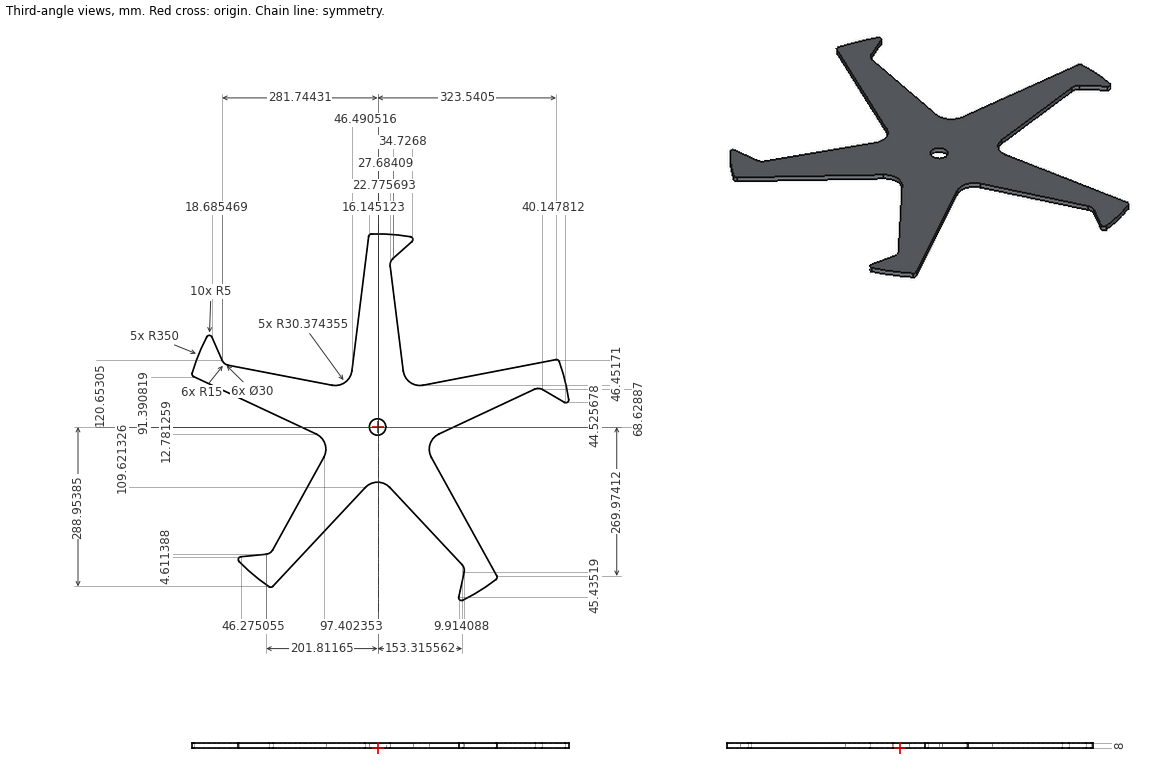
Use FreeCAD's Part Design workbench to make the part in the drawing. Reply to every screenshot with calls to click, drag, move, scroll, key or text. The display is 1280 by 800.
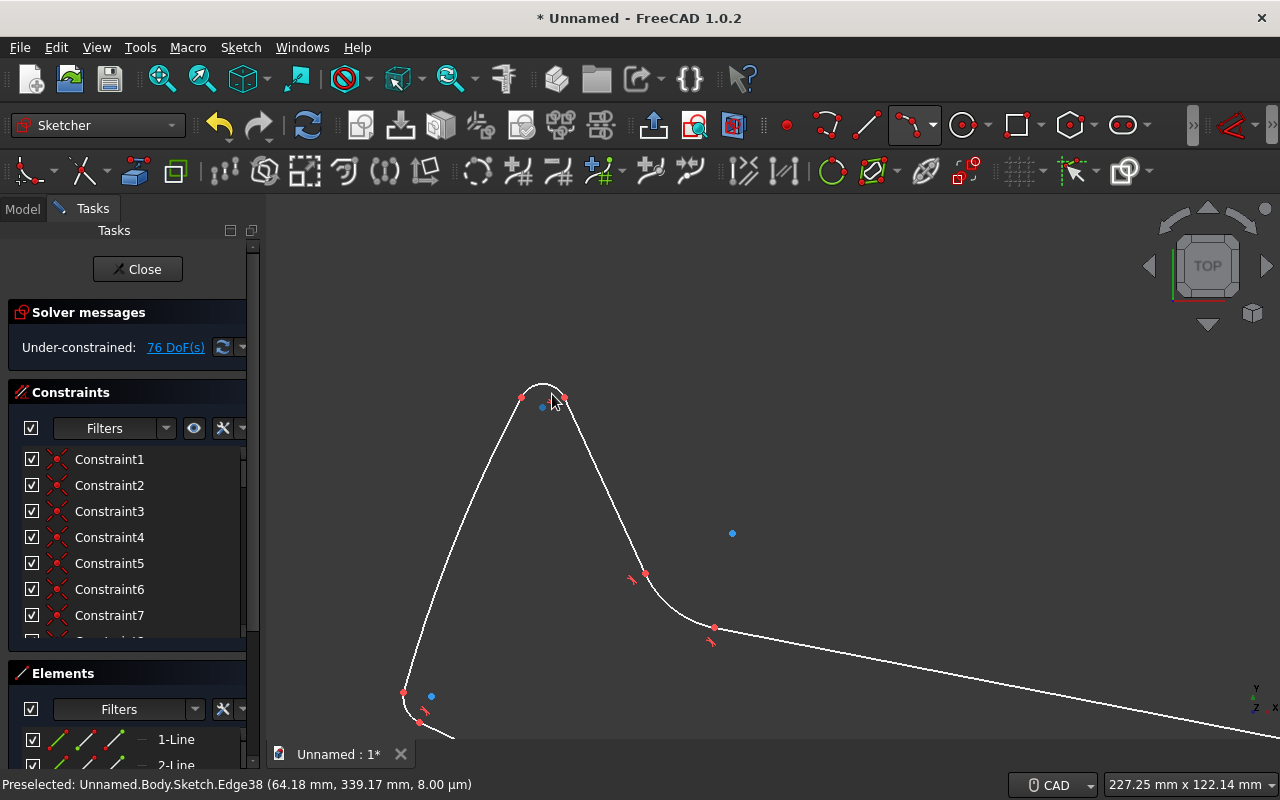
click(554, 387)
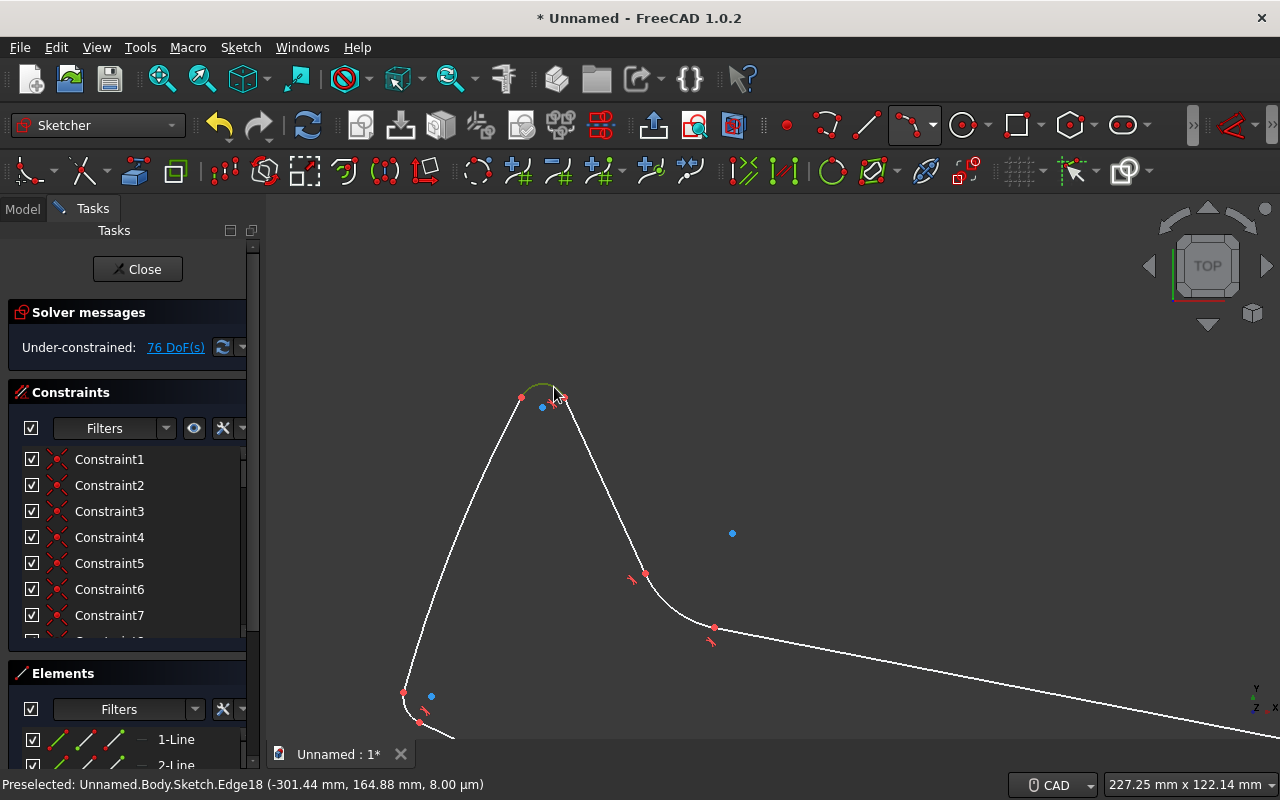
scroll(552, 394, down, 11)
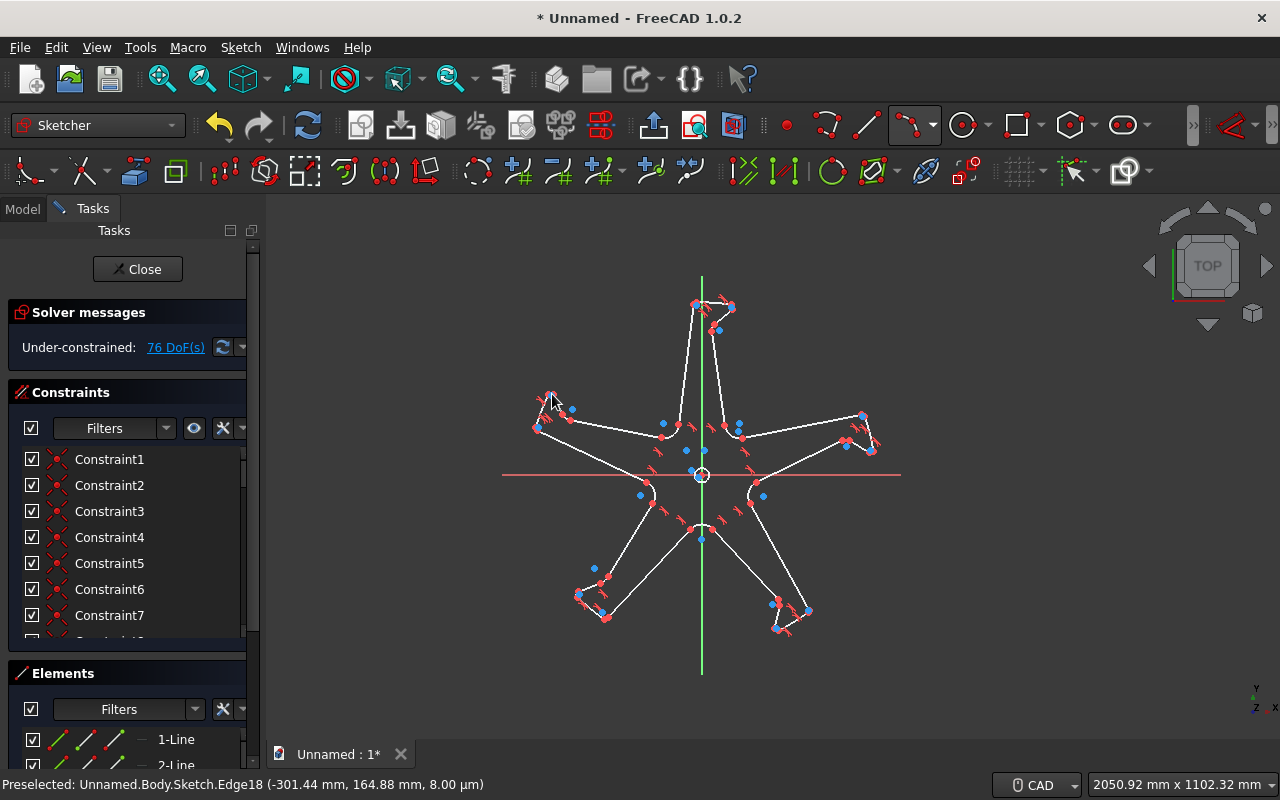
scroll(544, 404, up, 2)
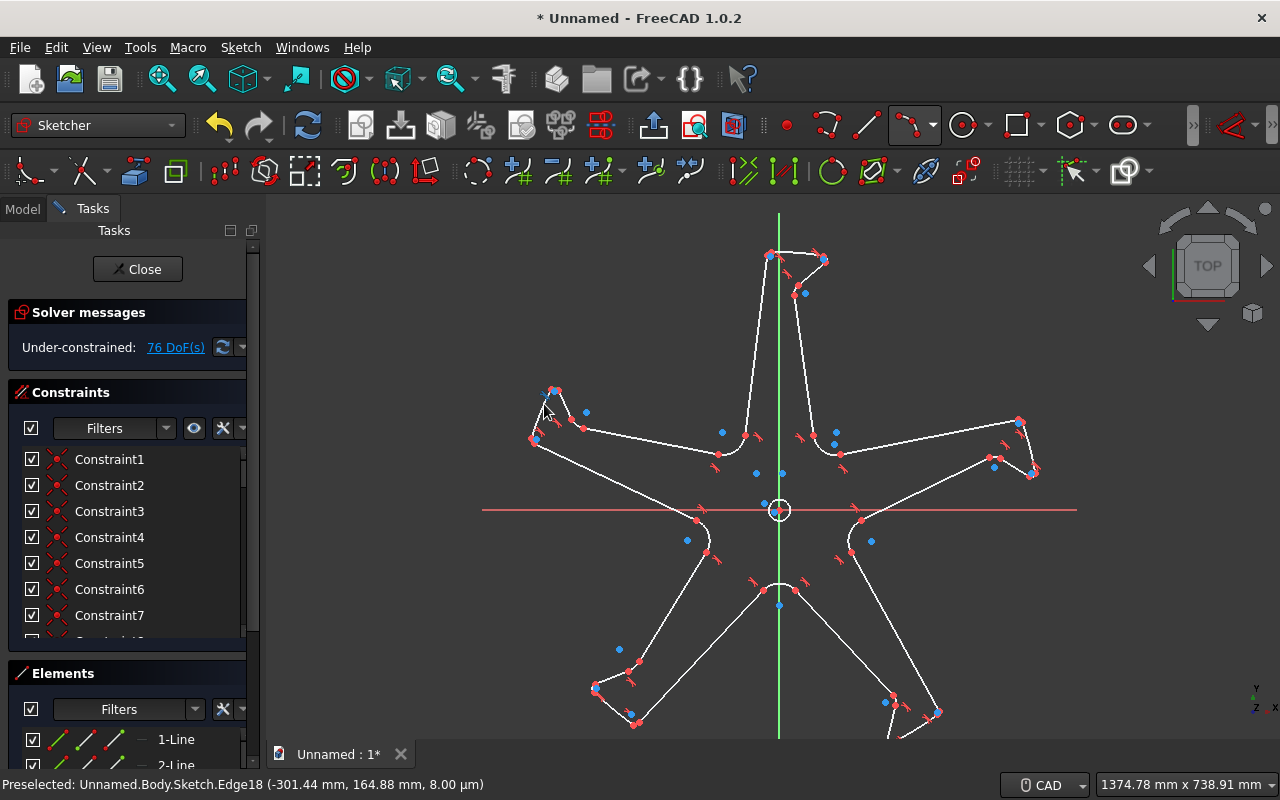
click(544, 404)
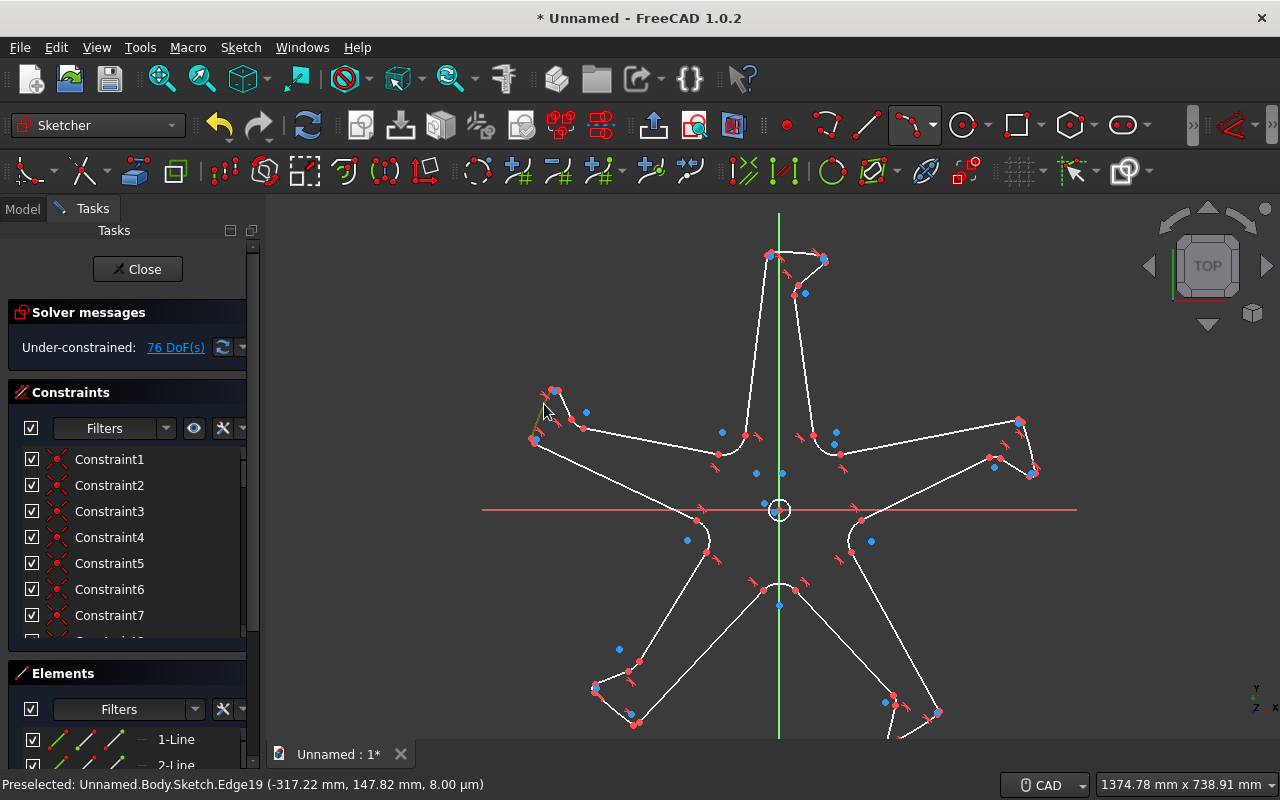
key(t)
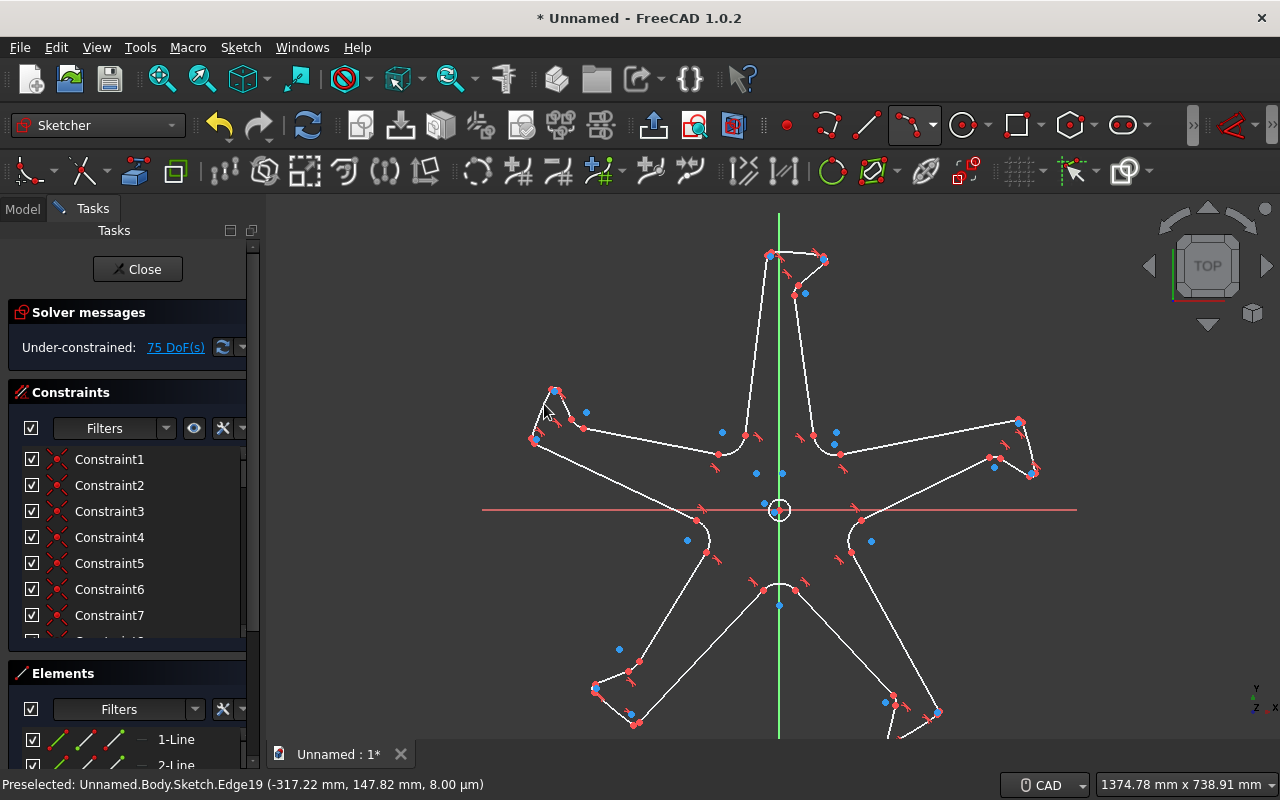
click(544, 404)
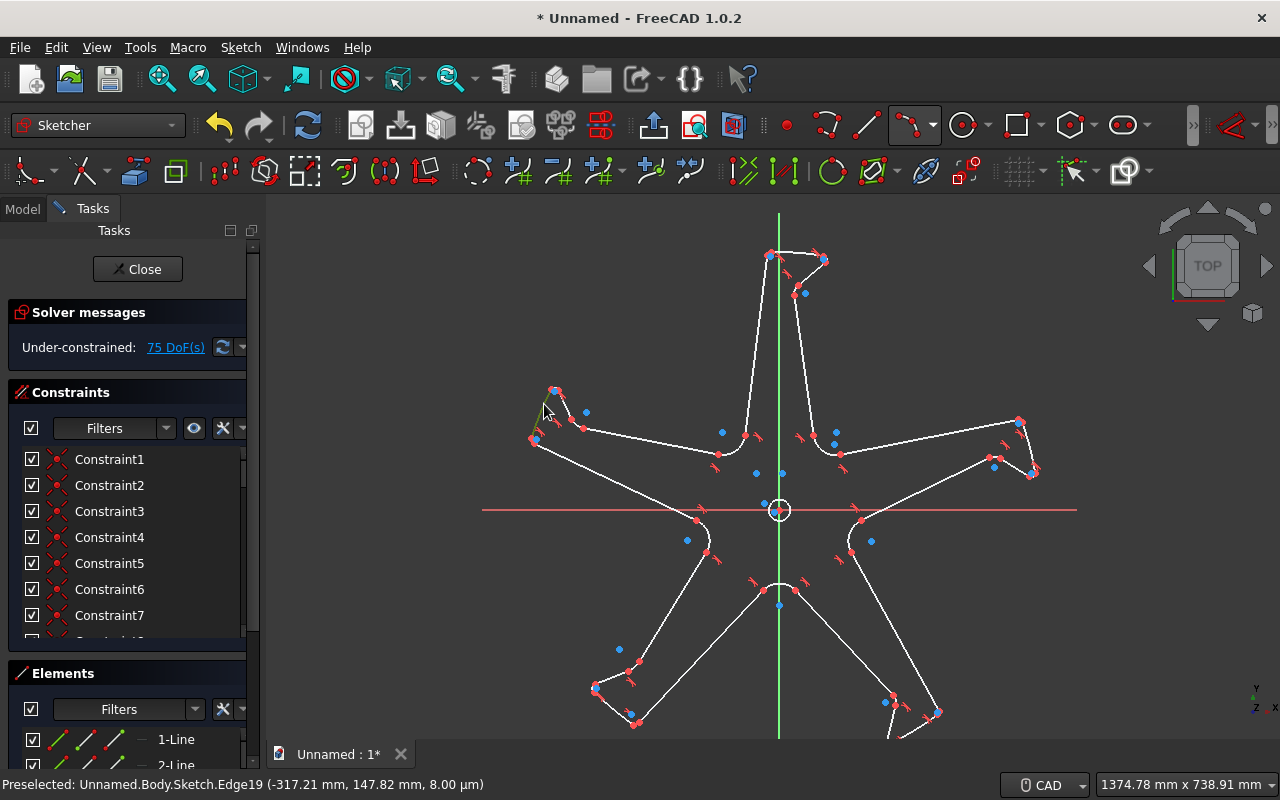
scroll(532, 442, up, 8)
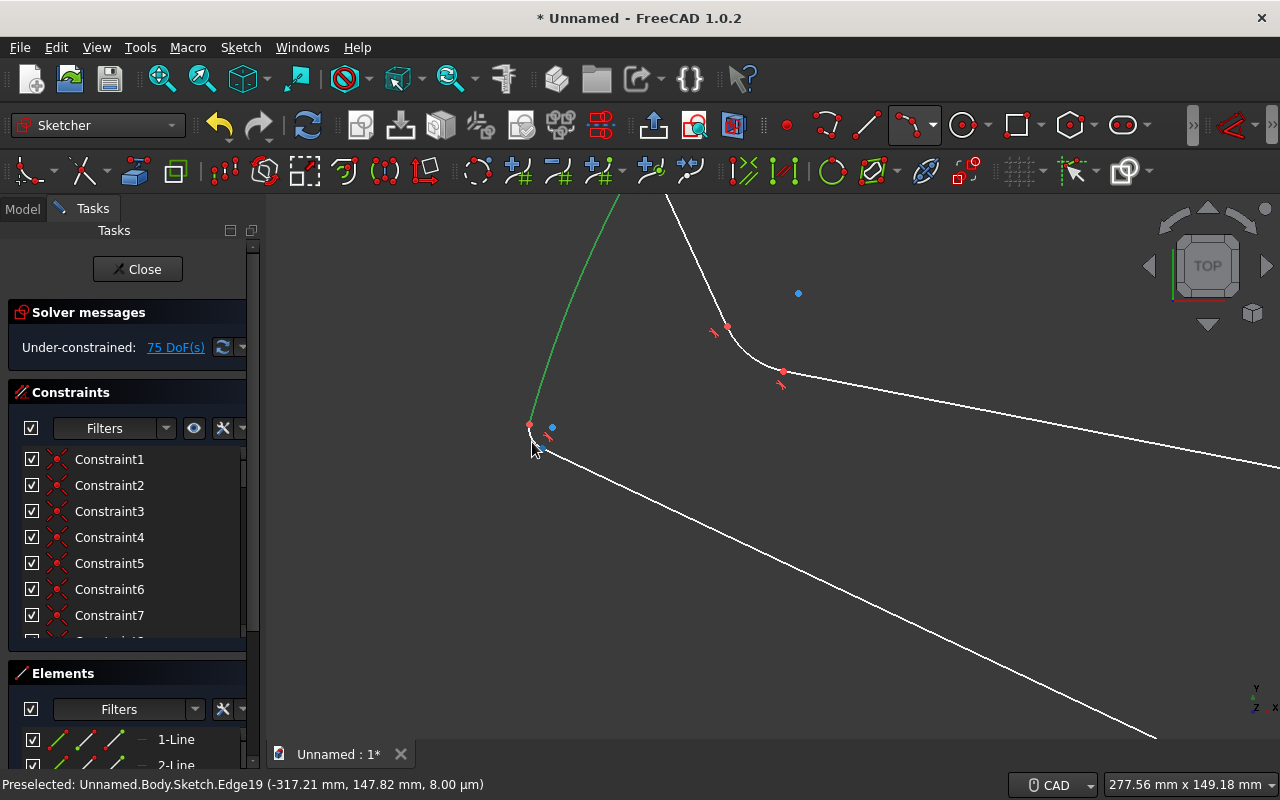
click(532, 438)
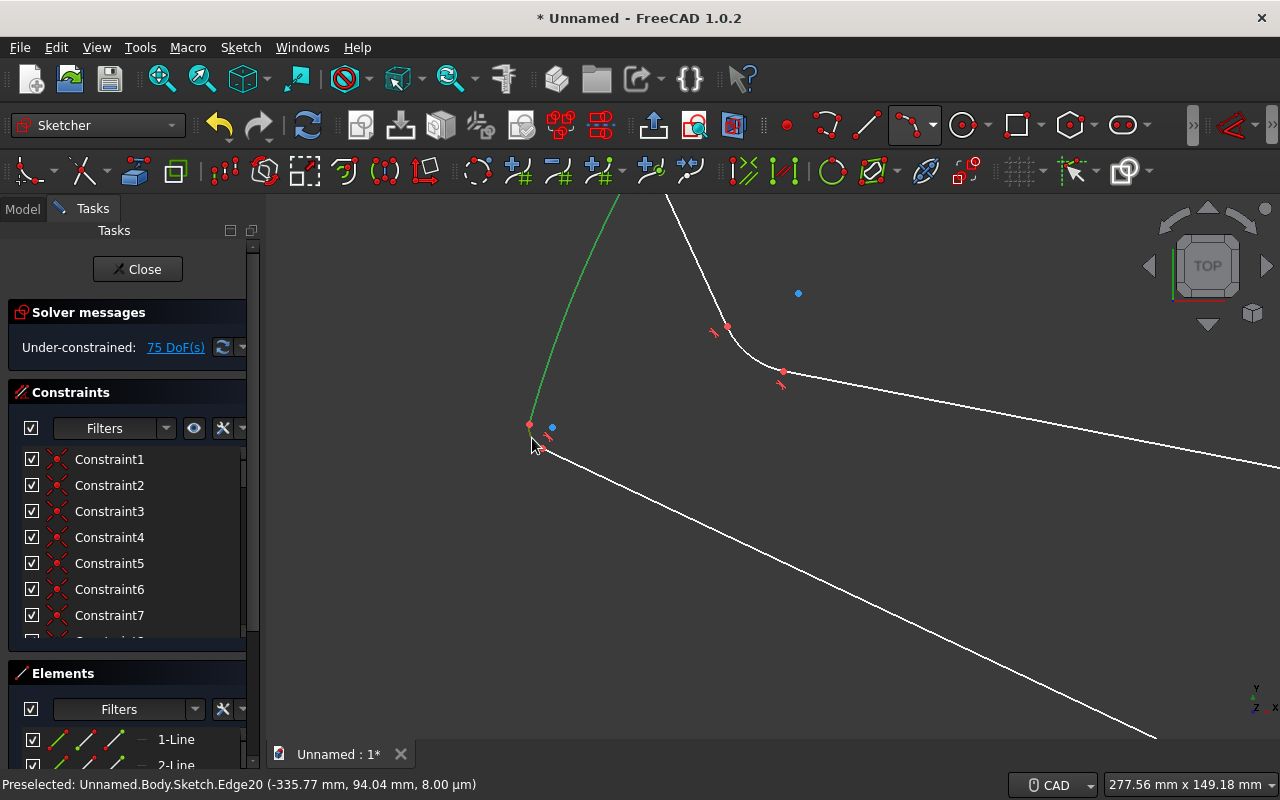
key(t)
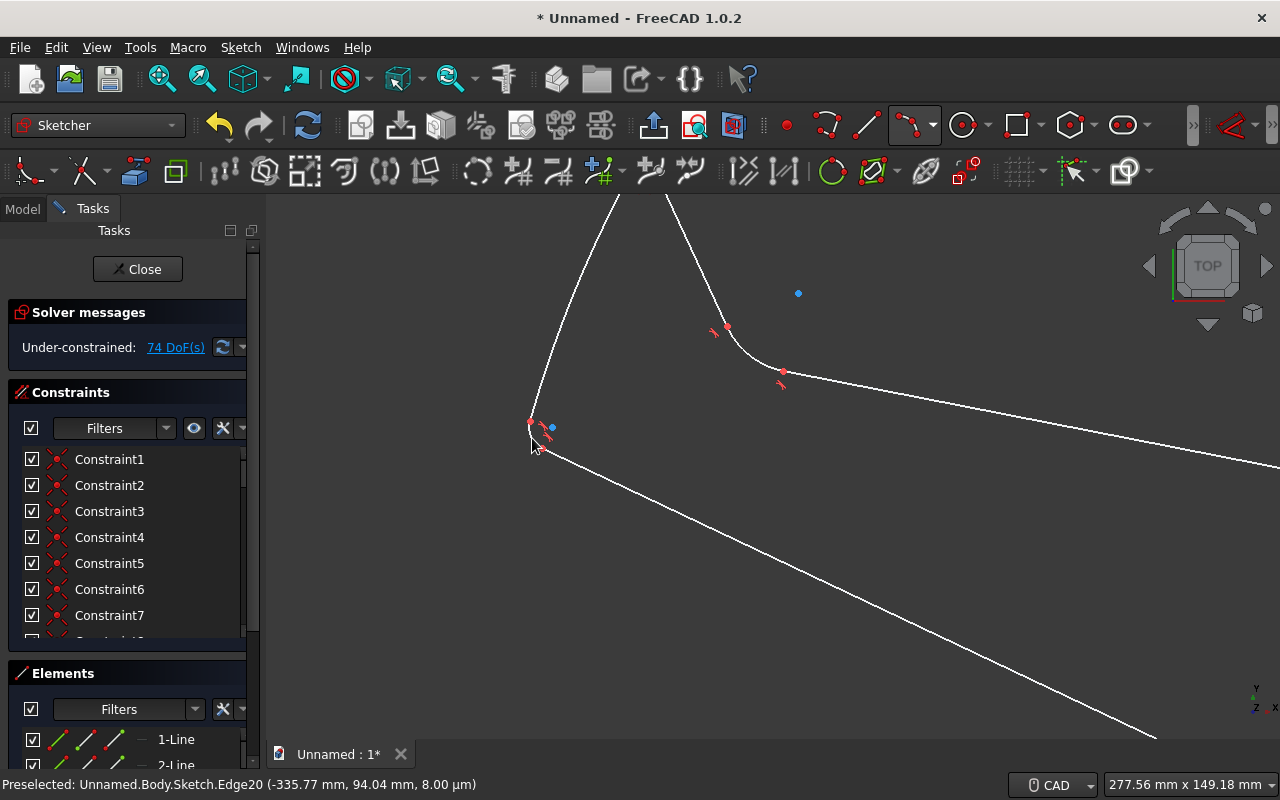
scroll(537, 428, down, 10)